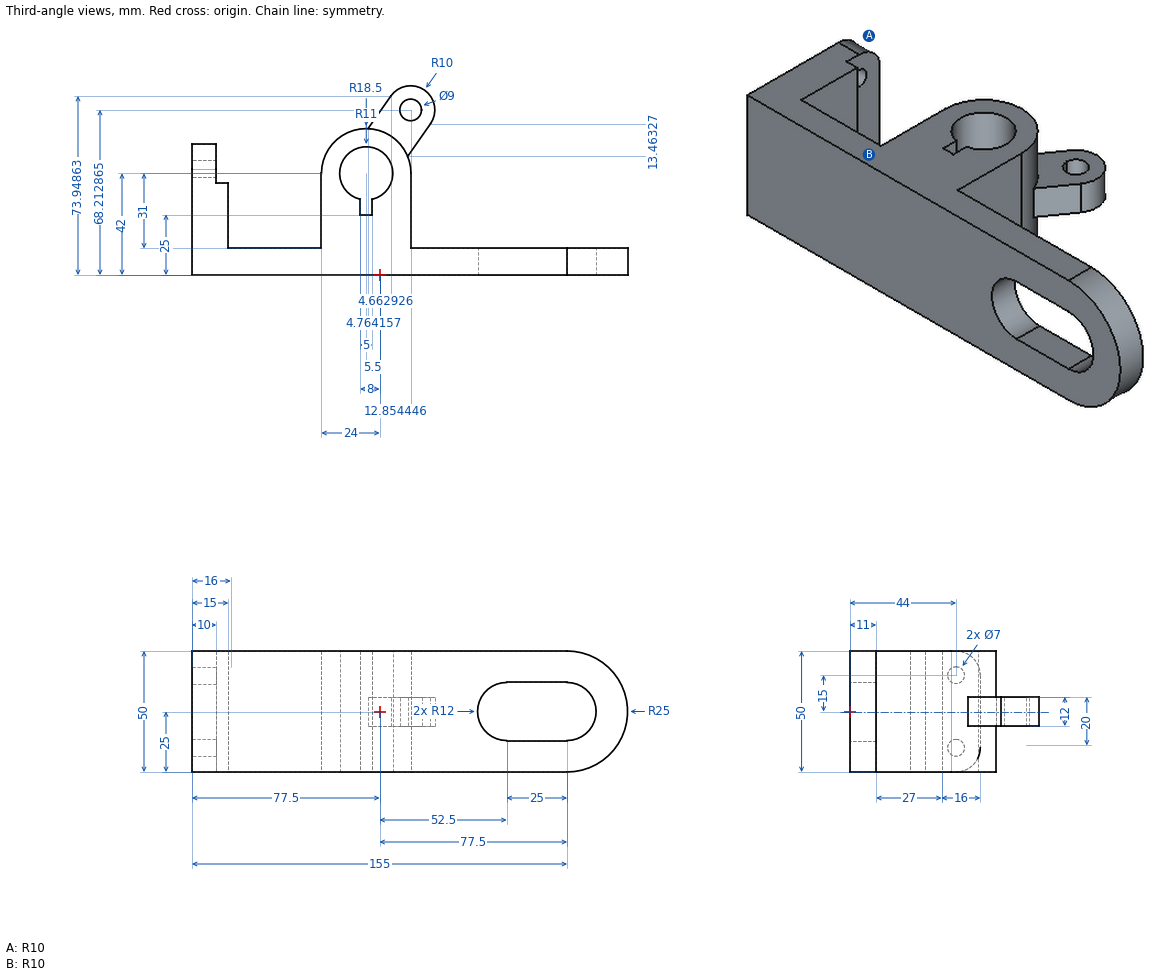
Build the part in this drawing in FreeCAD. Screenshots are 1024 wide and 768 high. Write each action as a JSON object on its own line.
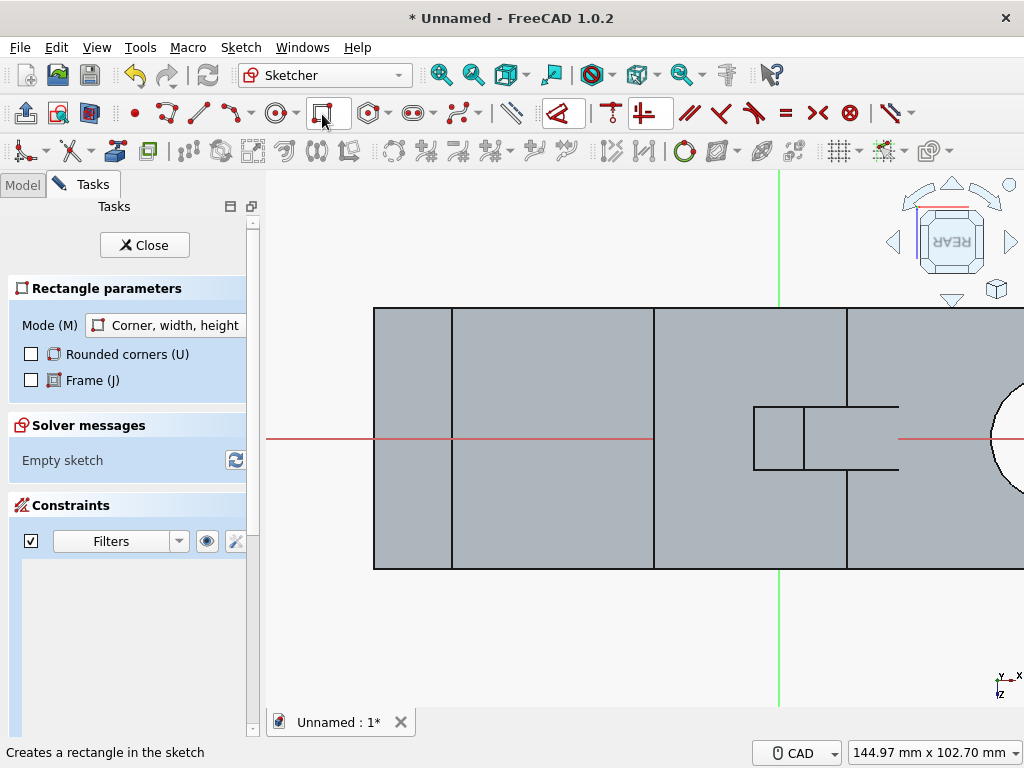
{"action": "left_click", "coordinate": [374, 308]}
{"action": "left_click", "coordinate": [426, 569]}
{"action": "key", "text": "Escape"}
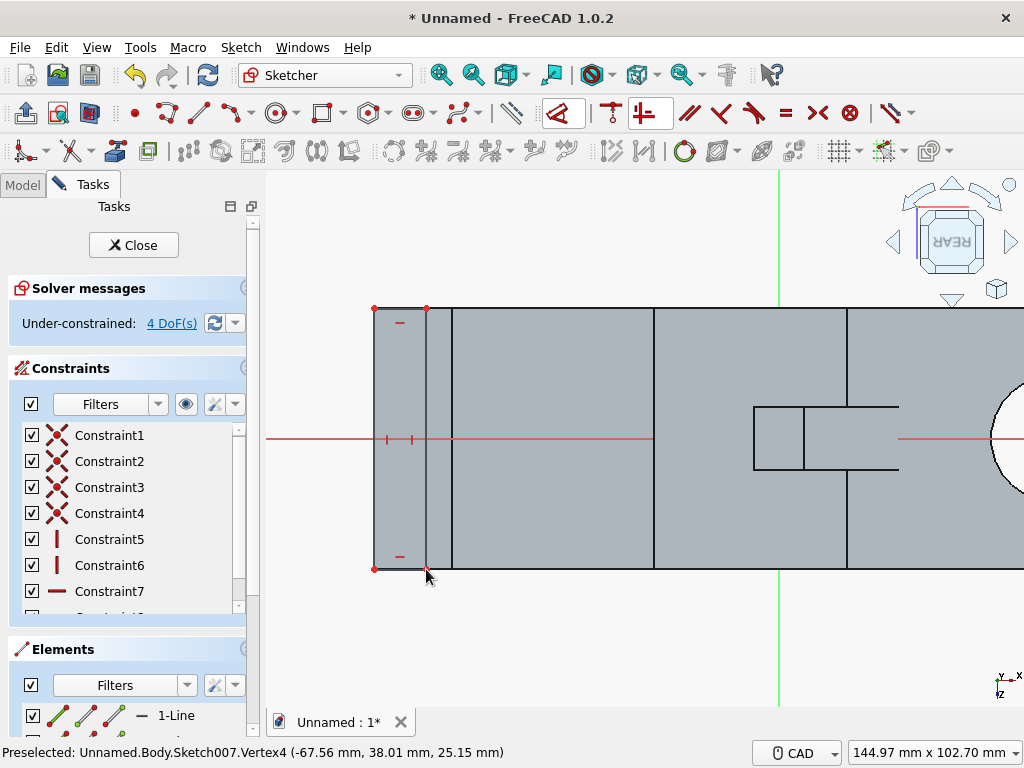
{"action": "left_click", "coordinate": [374, 387]}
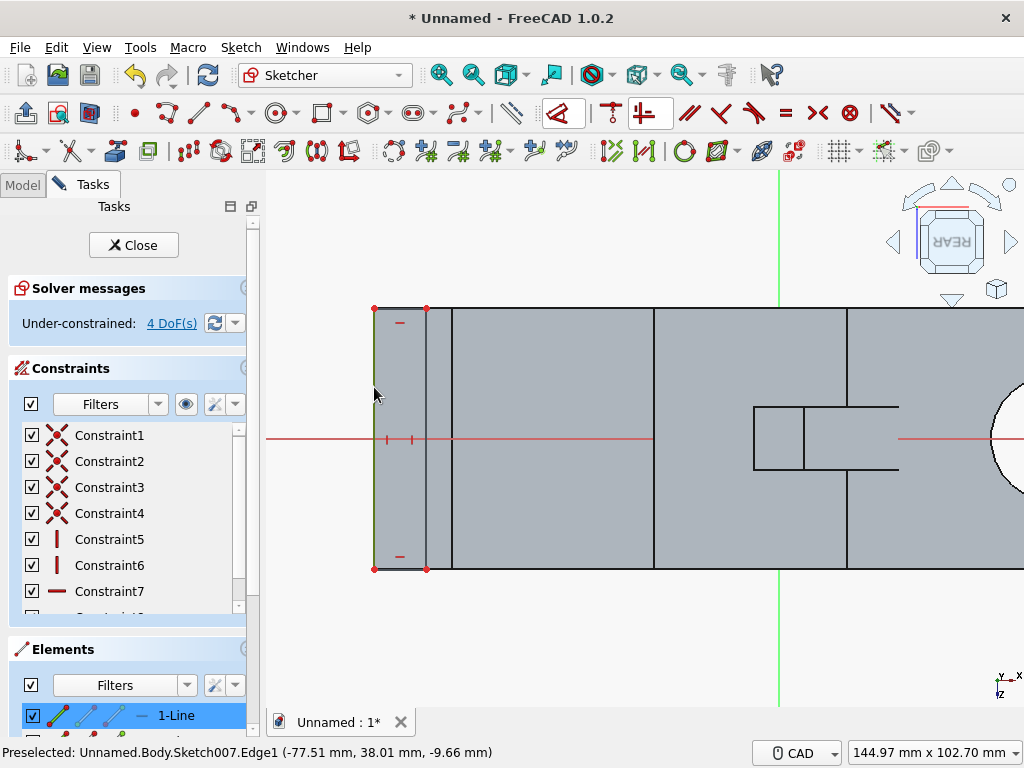
{"action": "left_click", "coordinate": [580, 114]}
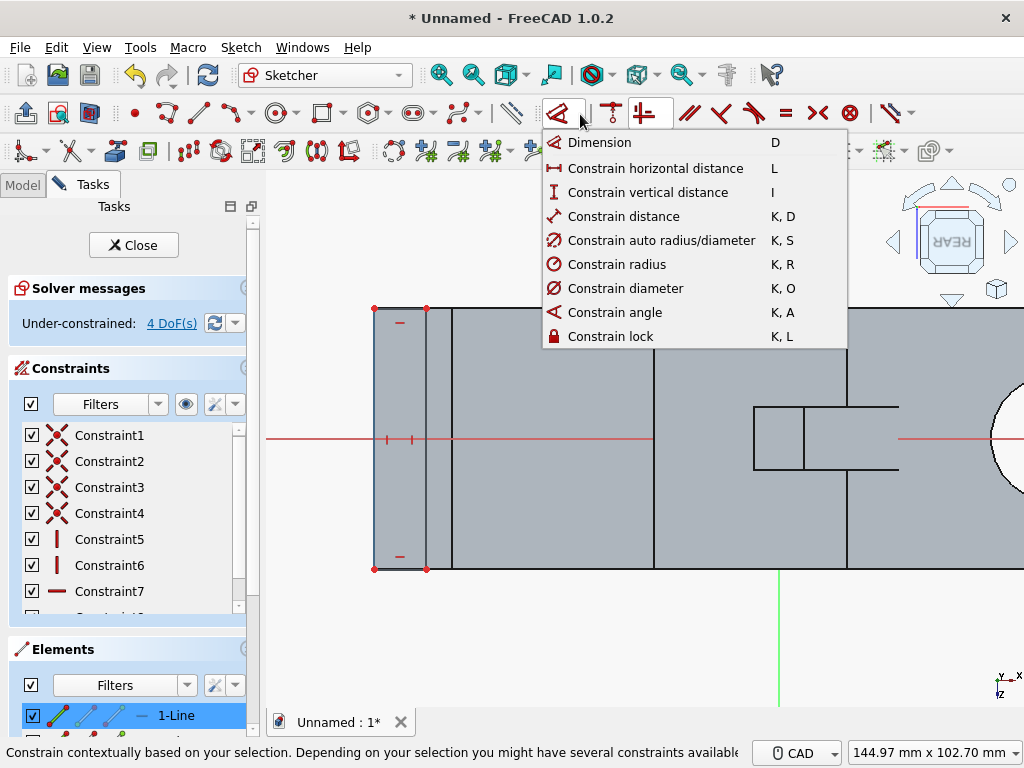
{"action": "left_click", "coordinate": [695, 192]}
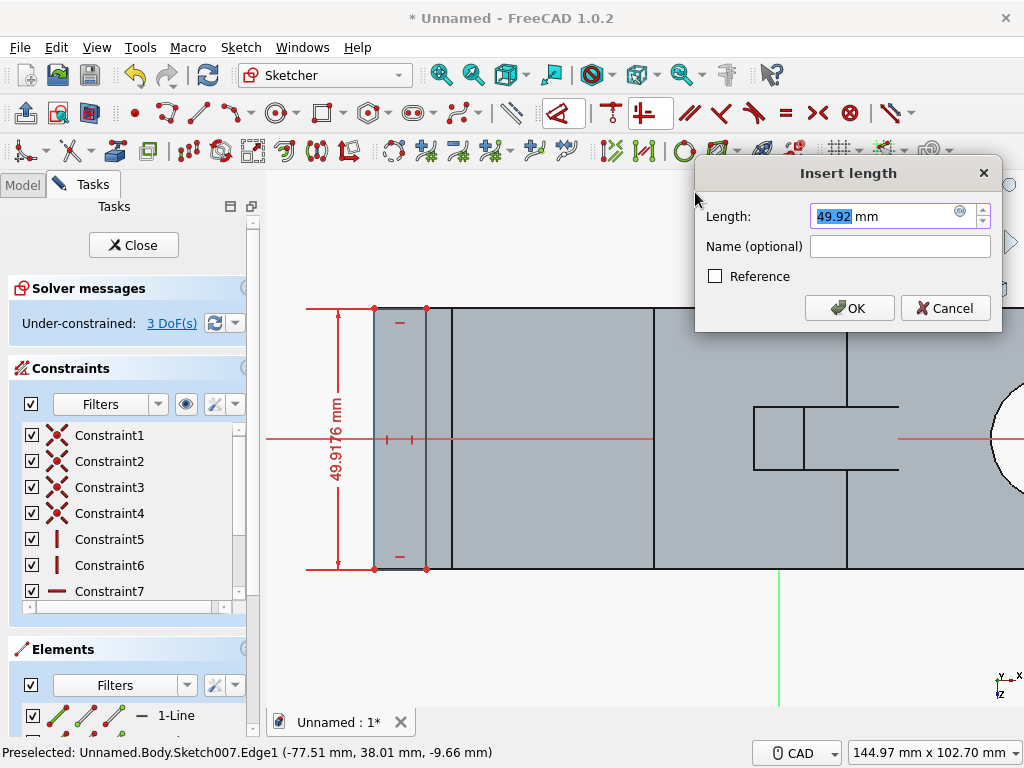
{"action": "type", "text": "50"}
{"action": "key", "text": "Return"}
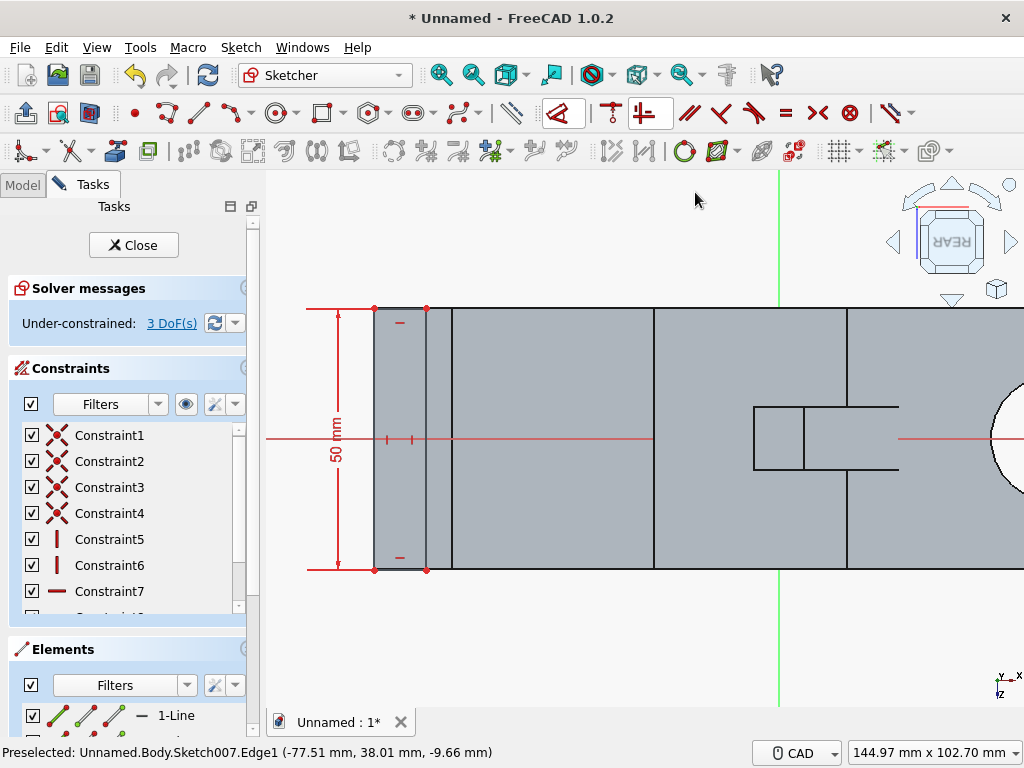
{"action": "left_click", "coordinate": [390, 570]}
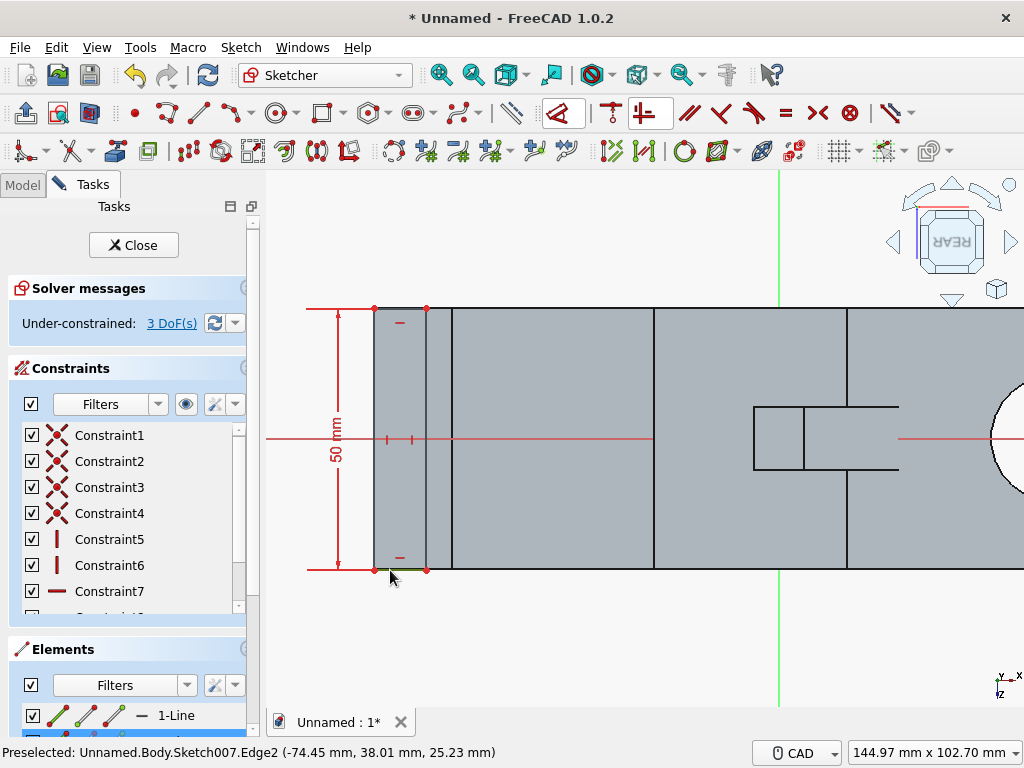
{"action": "left_click", "coordinate": [580, 114]}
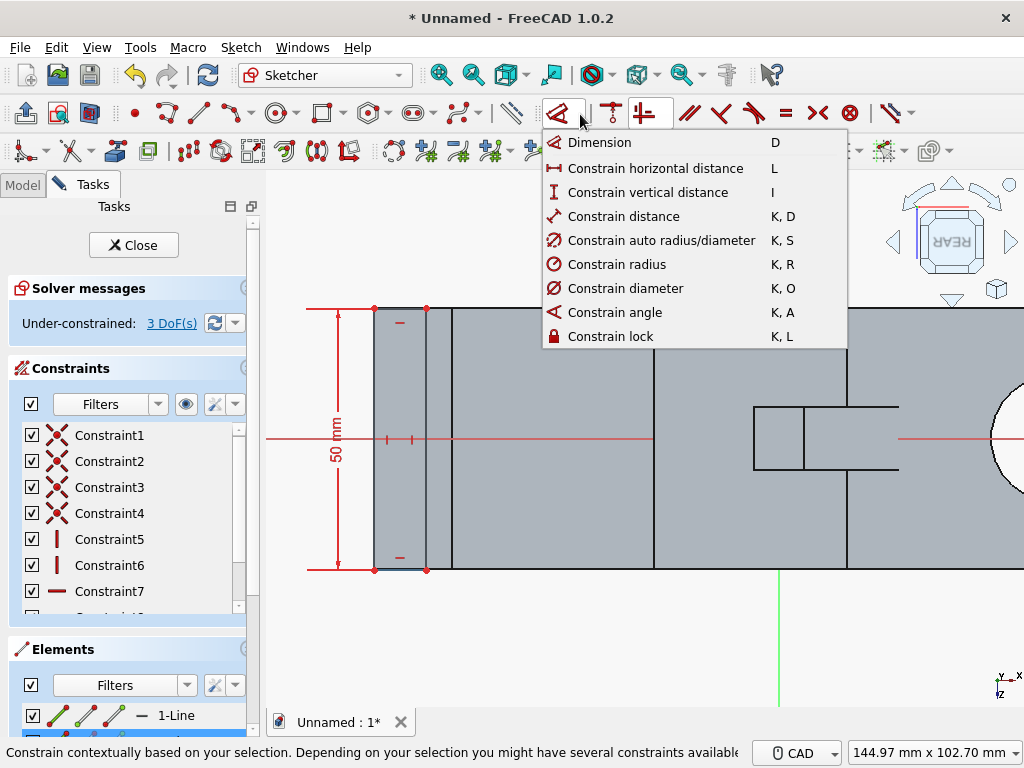
{"action": "left_click", "coordinate": [695, 168]}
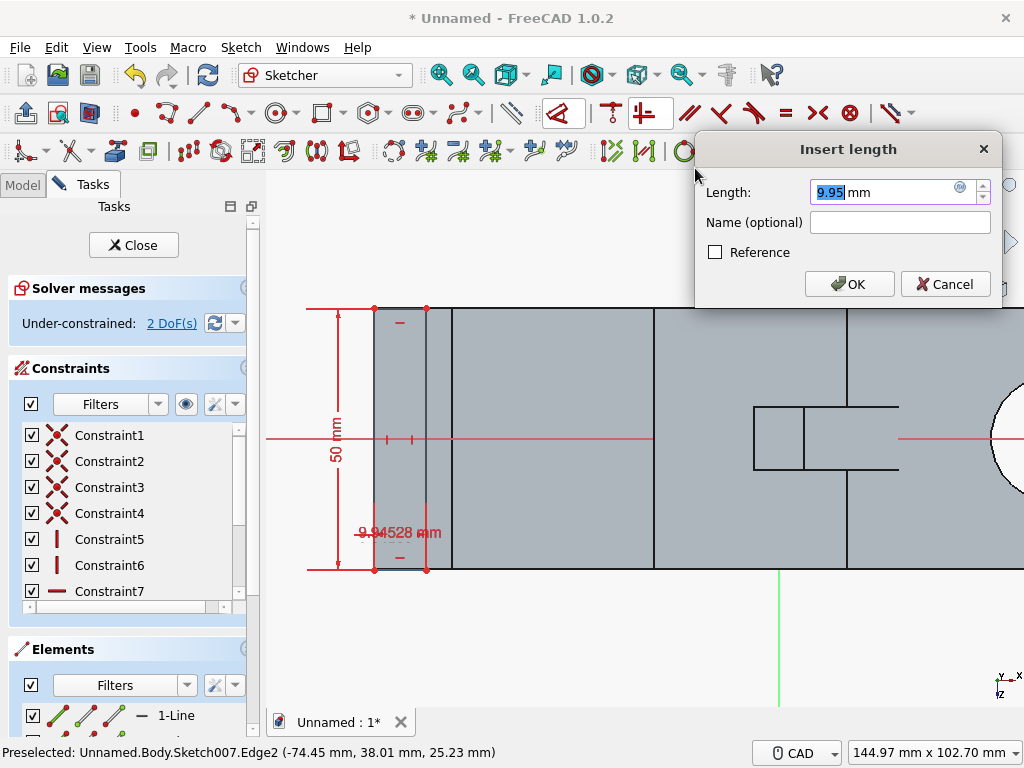
{"action": "type", "text": "10"}
{"action": "key", "text": "Return"}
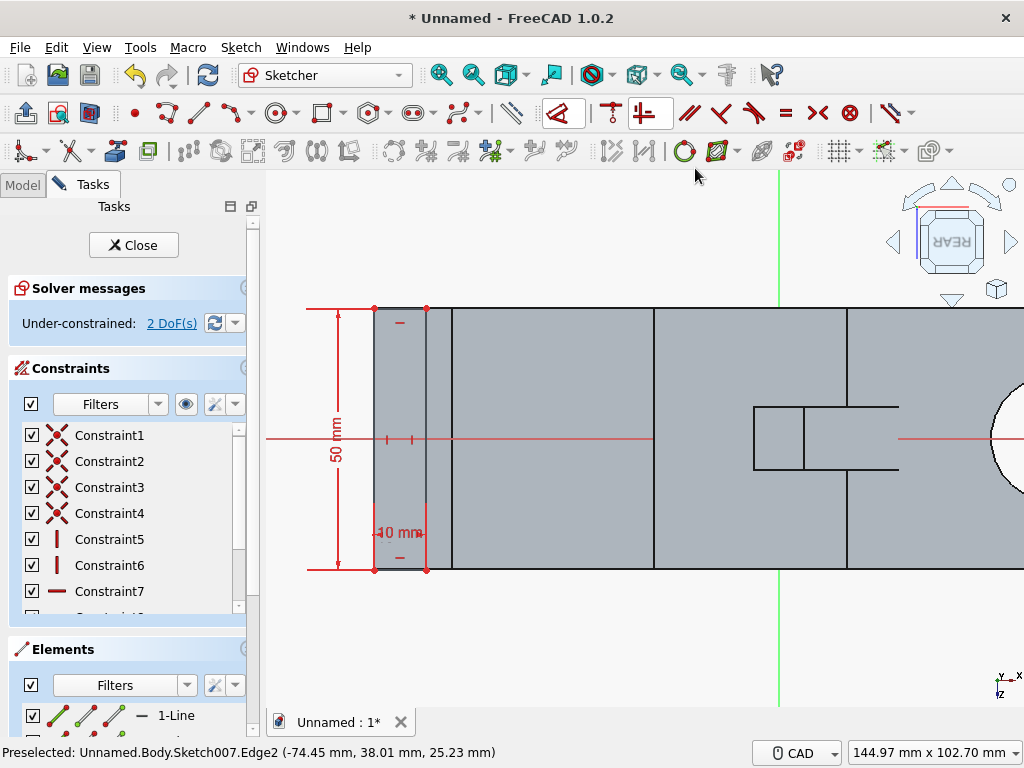
{"action": "left_click", "coordinate": [374, 309]}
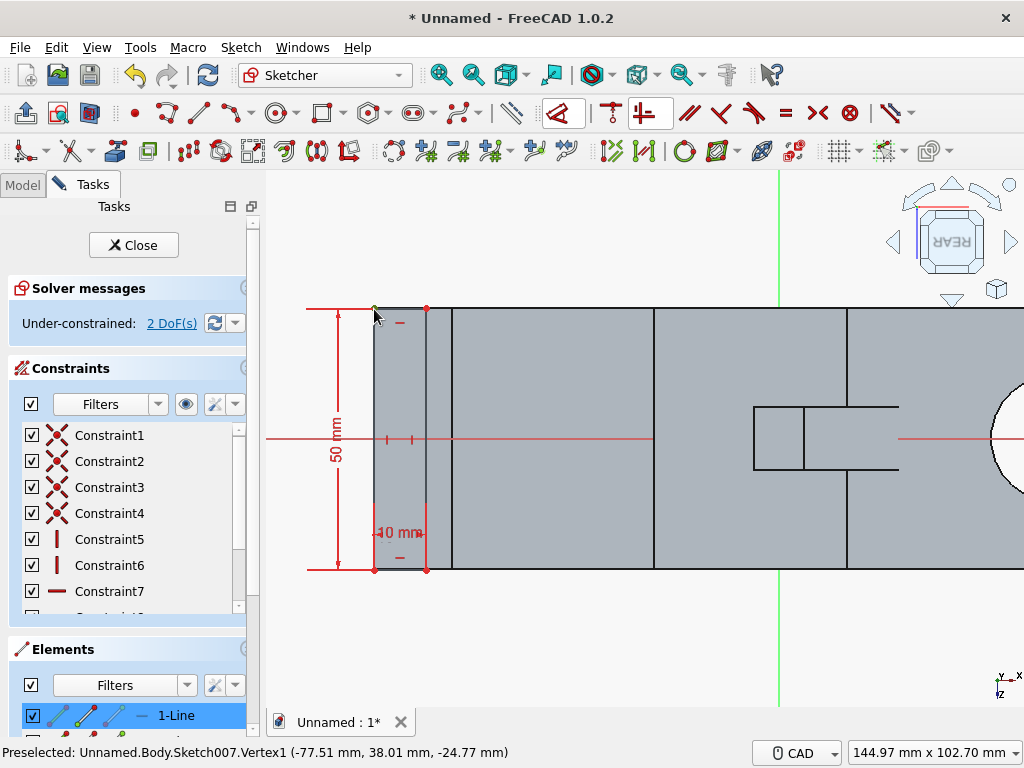
{"action": "key", "text": "i"}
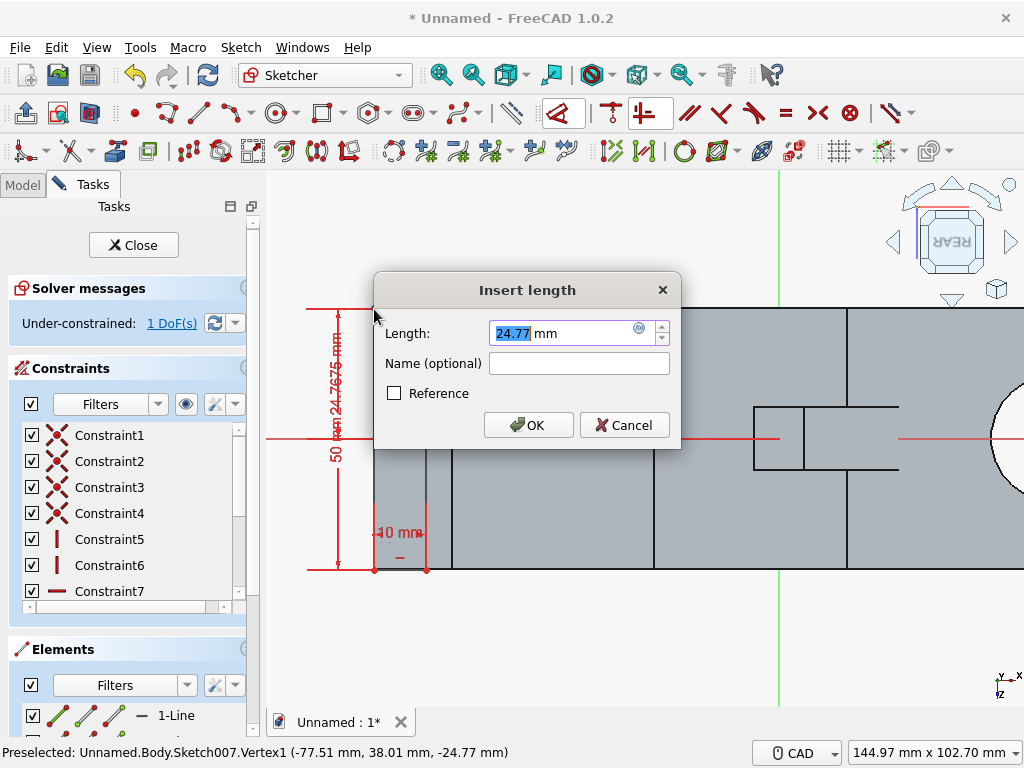
{"action": "type", "text": "25"}
{"action": "key", "text": "Return"}